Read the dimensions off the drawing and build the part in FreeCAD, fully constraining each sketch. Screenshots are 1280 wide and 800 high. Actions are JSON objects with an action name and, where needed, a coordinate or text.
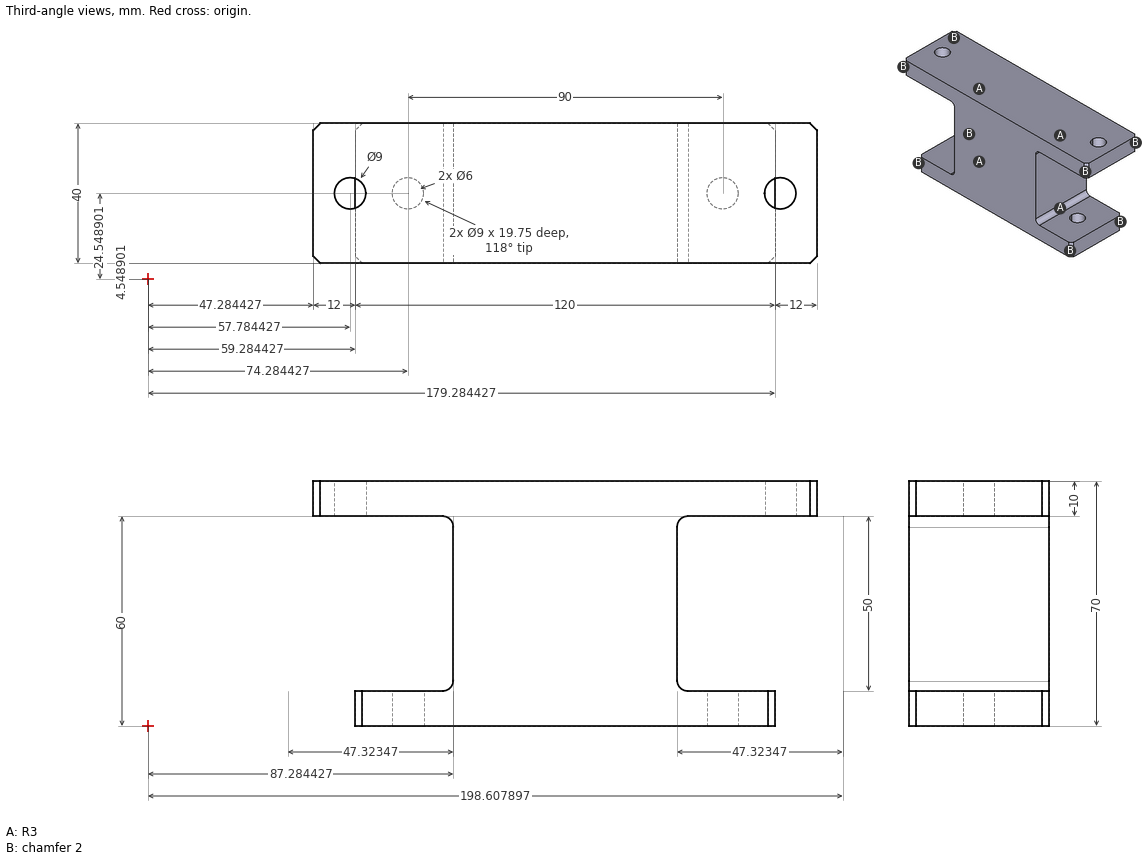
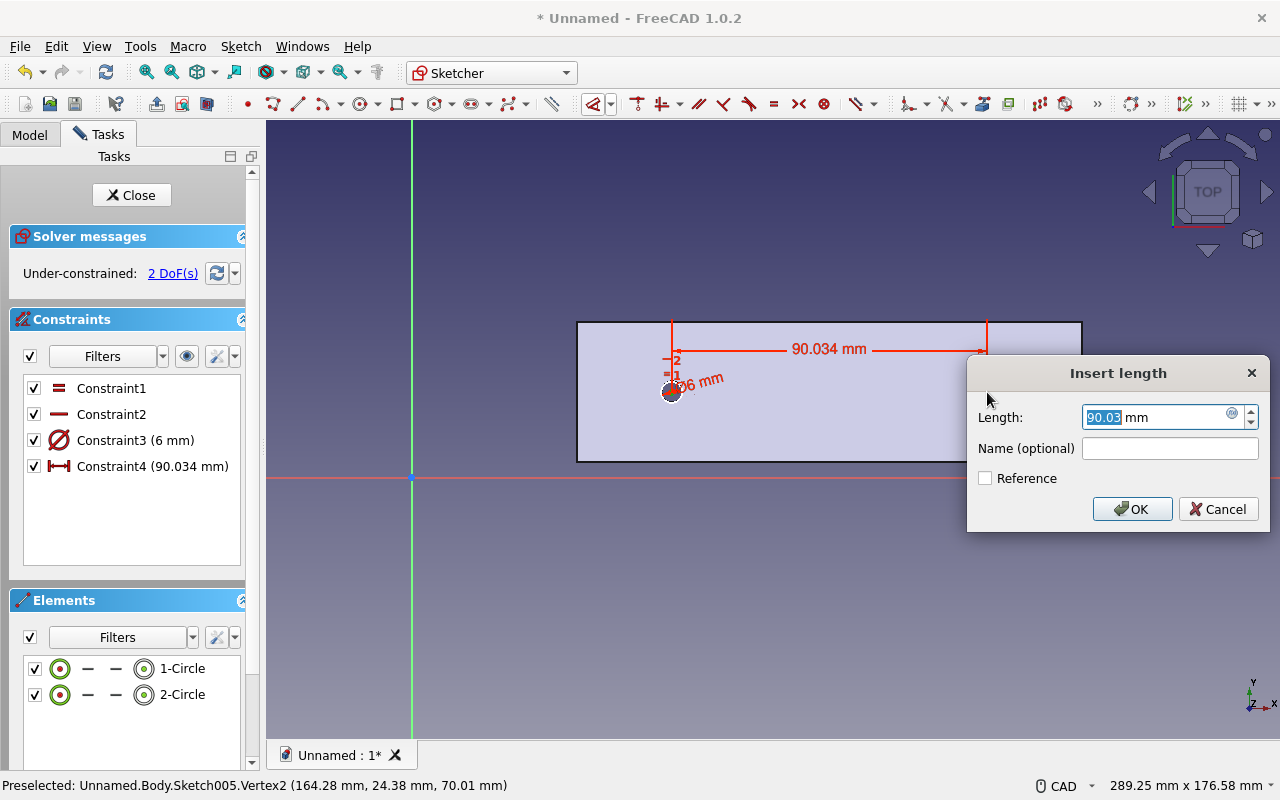
{"action": "type", "text": "90"}
{"action": "key", "text": "Return"}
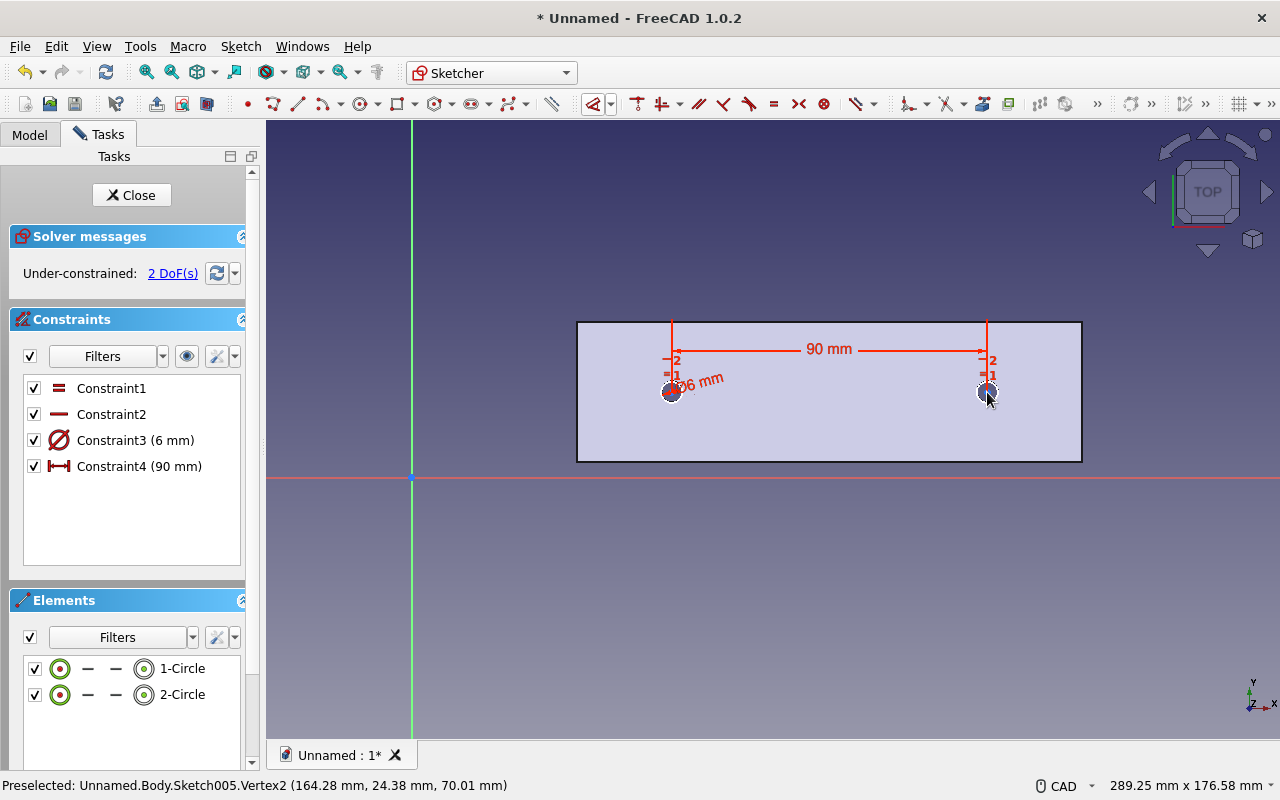
{"action": "left_click", "coordinate": [672, 392]}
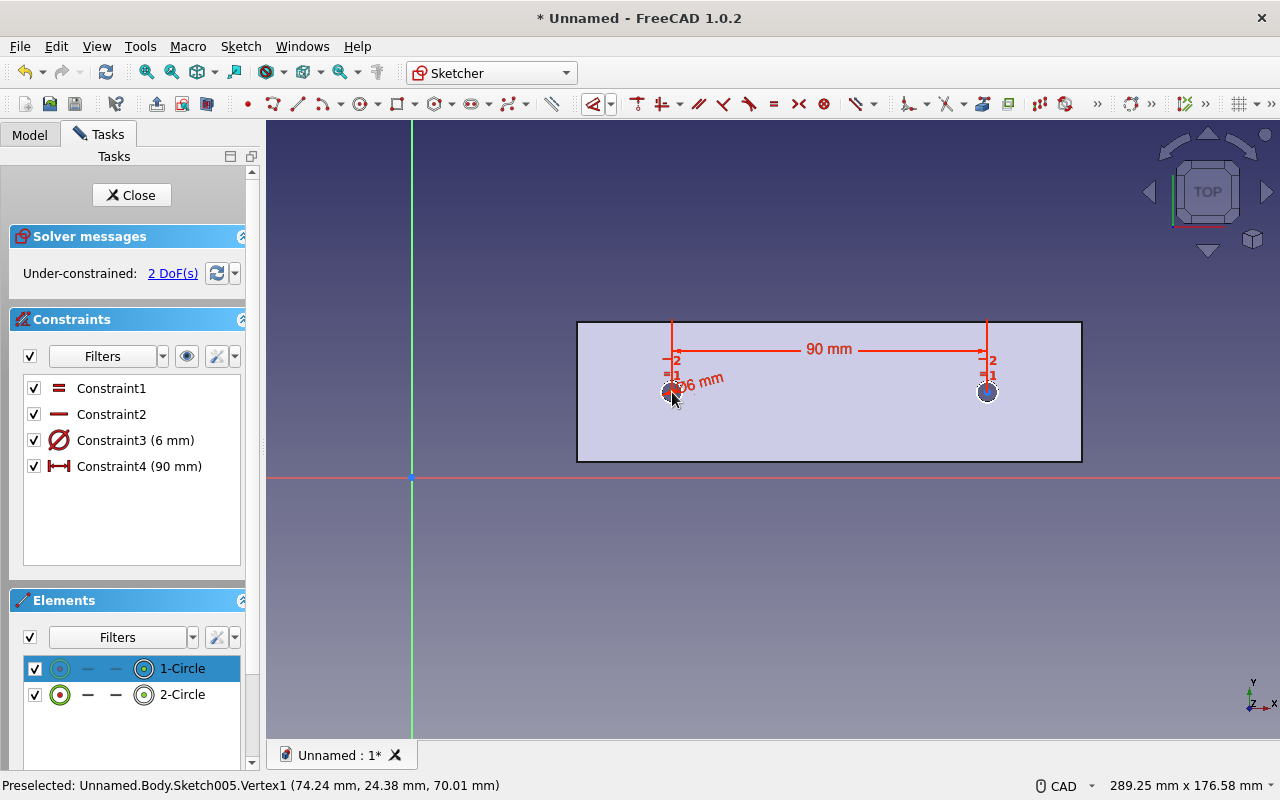
{"action": "key", "text": "l"}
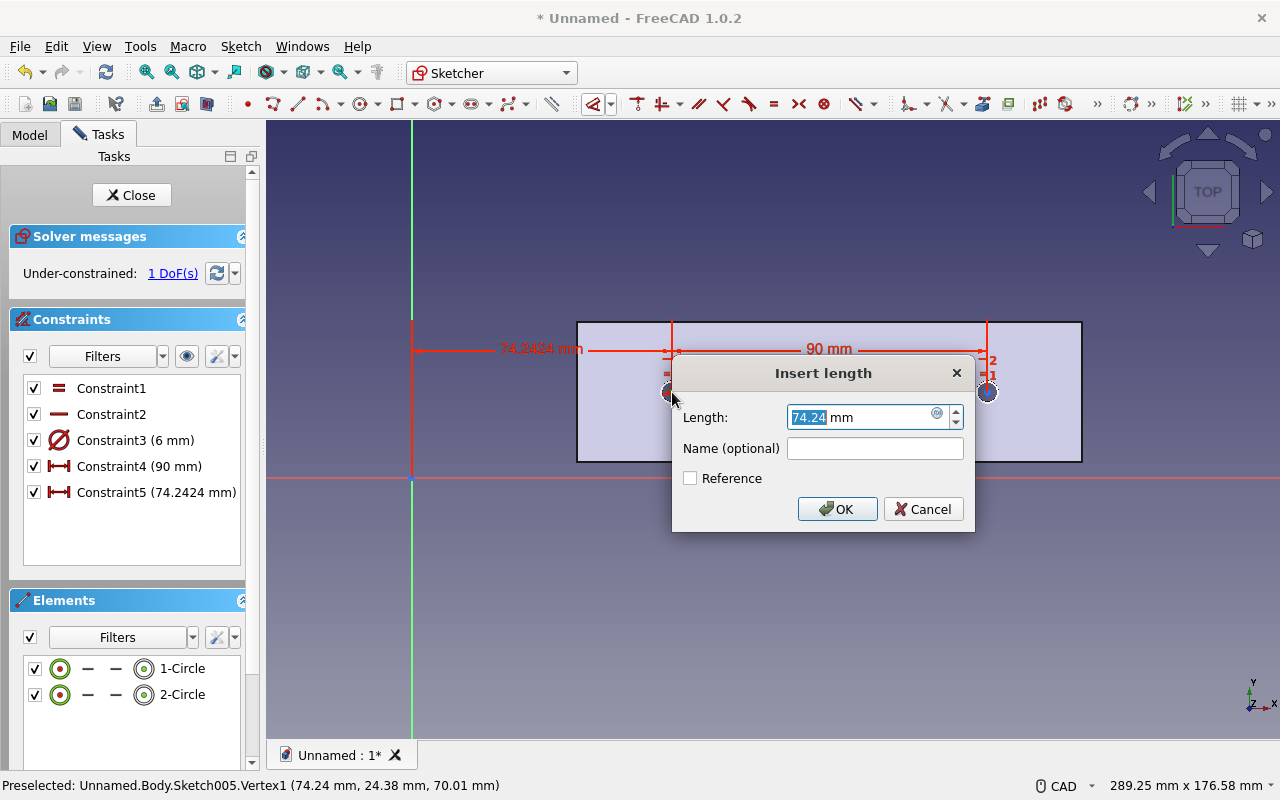
{"action": "type", "text": "74.284427"}
{"action": "key", "text": "Return"}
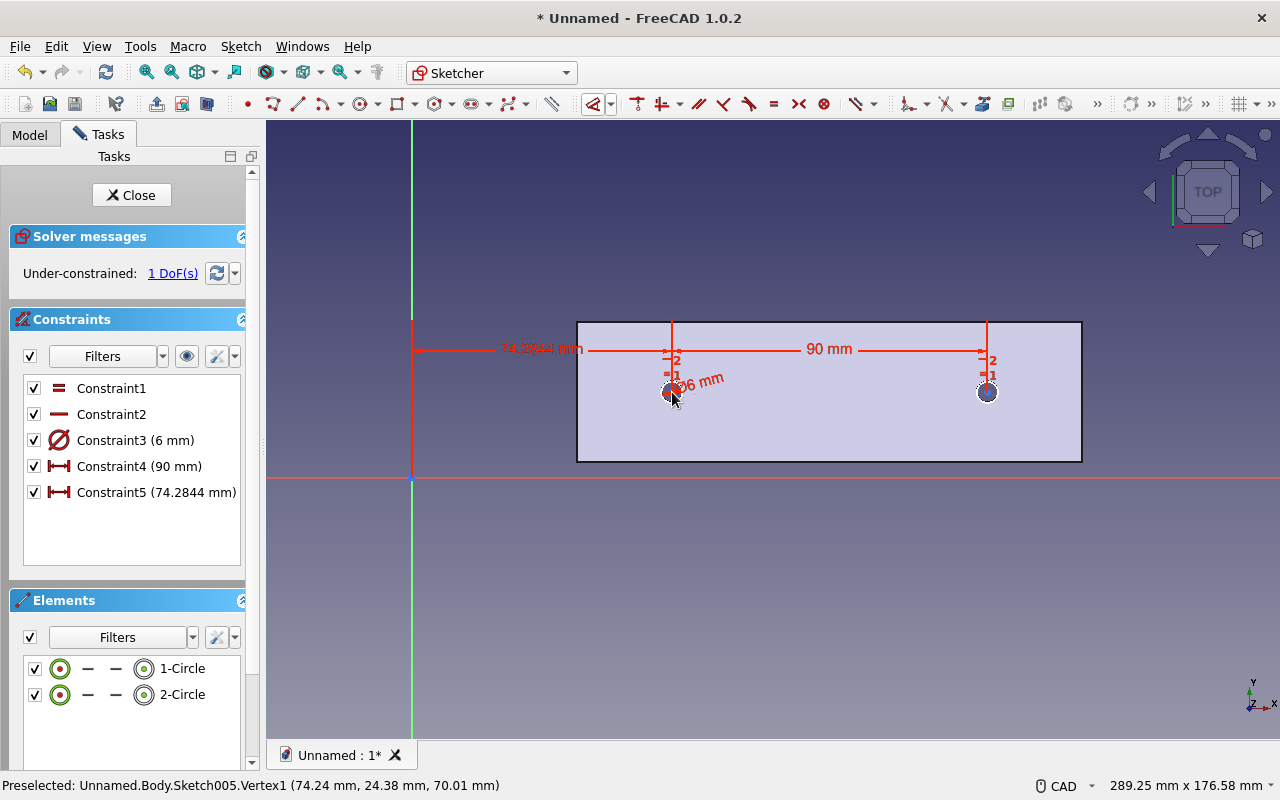
{"action": "left_click", "coordinate": [672, 392]}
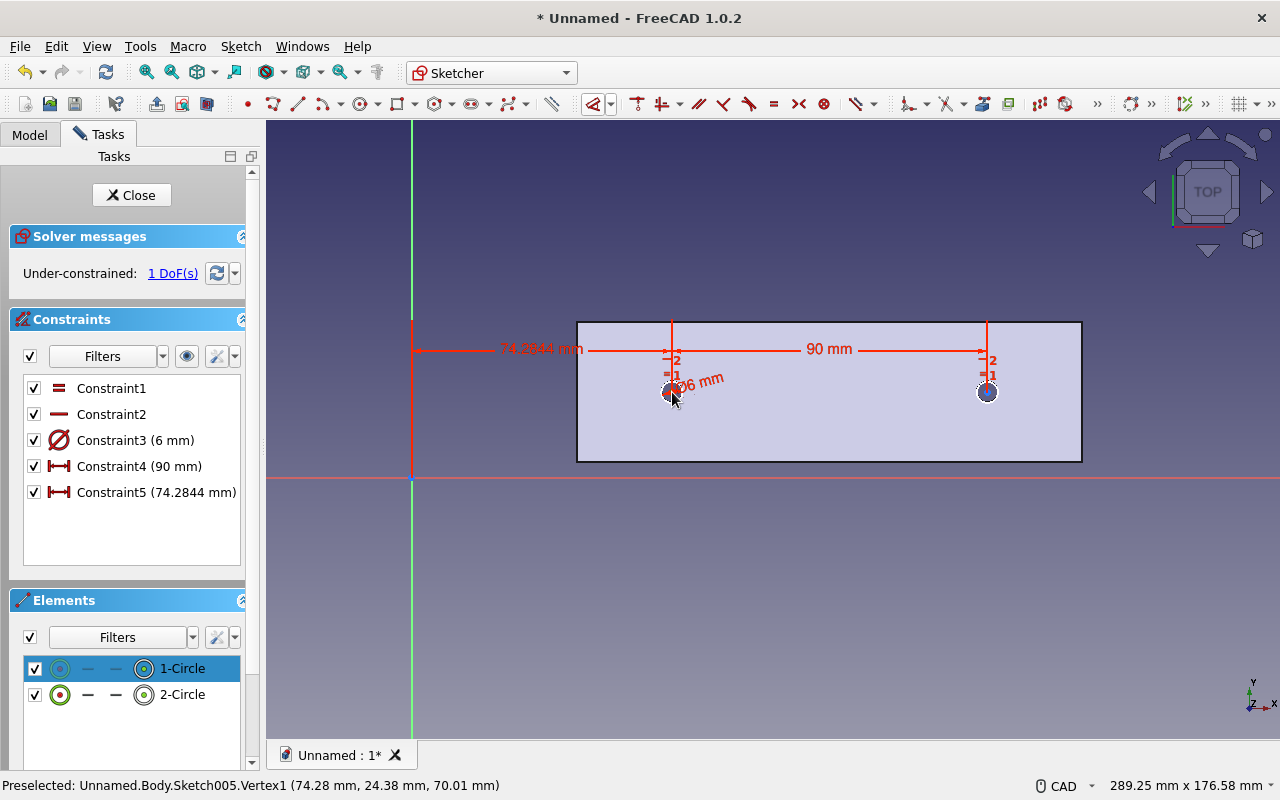
{"action": "key", "text": "i"}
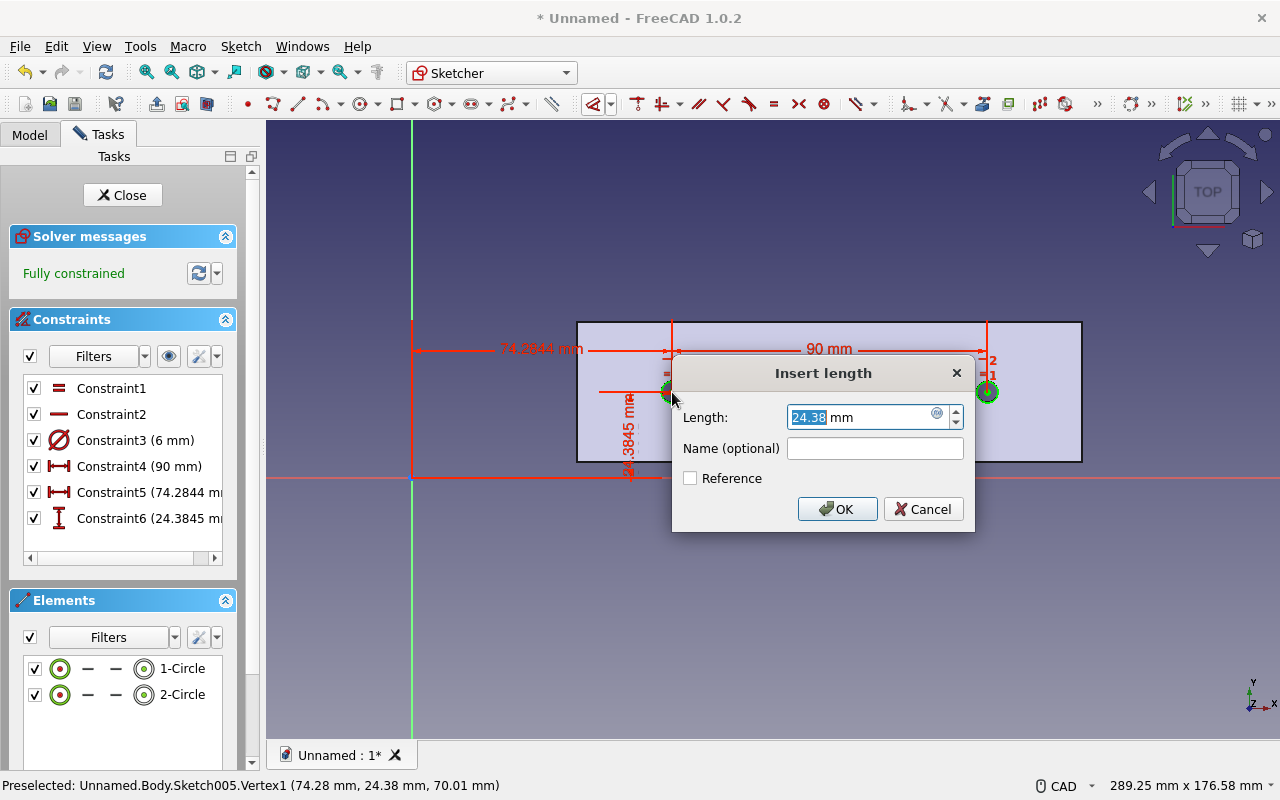
{"action": "type", "text": "24.548901"}
{"action": "key", "text": "Return"}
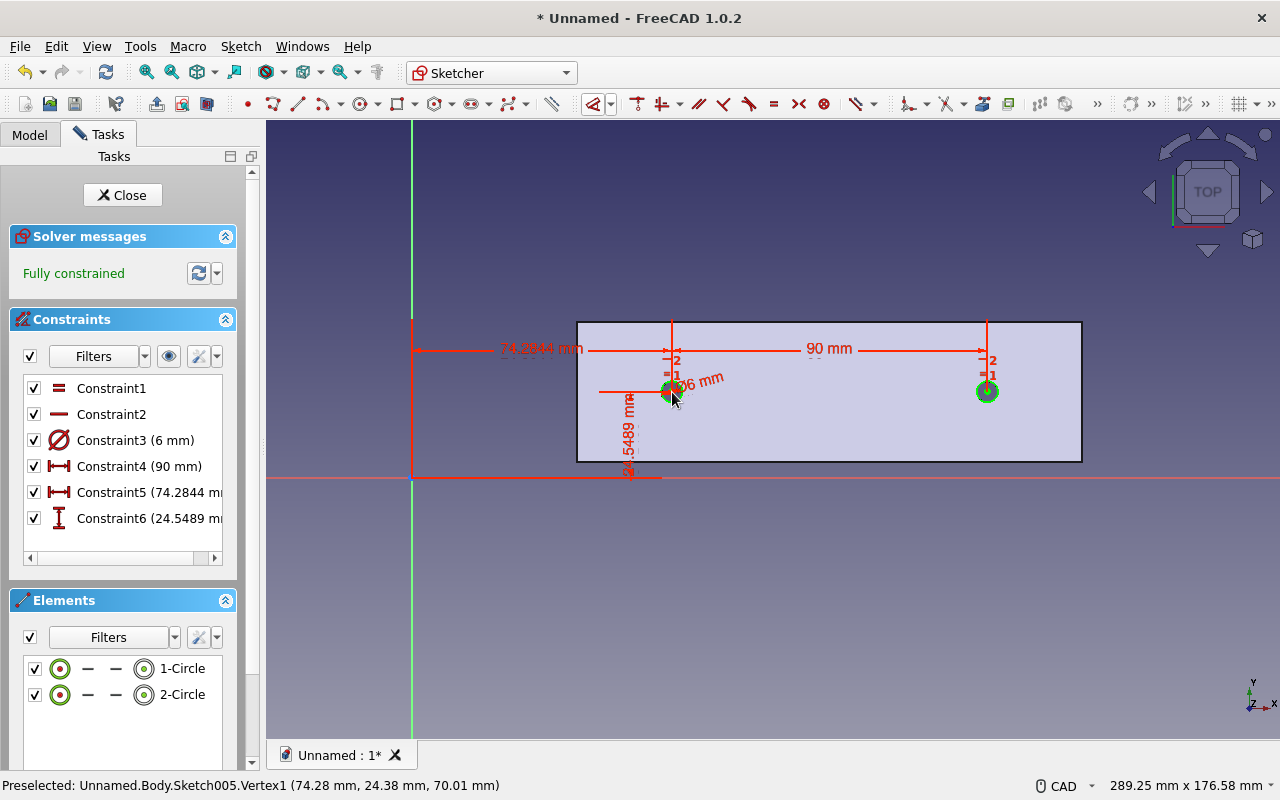
{"action": "left_click", "coordinate": [123, 195]}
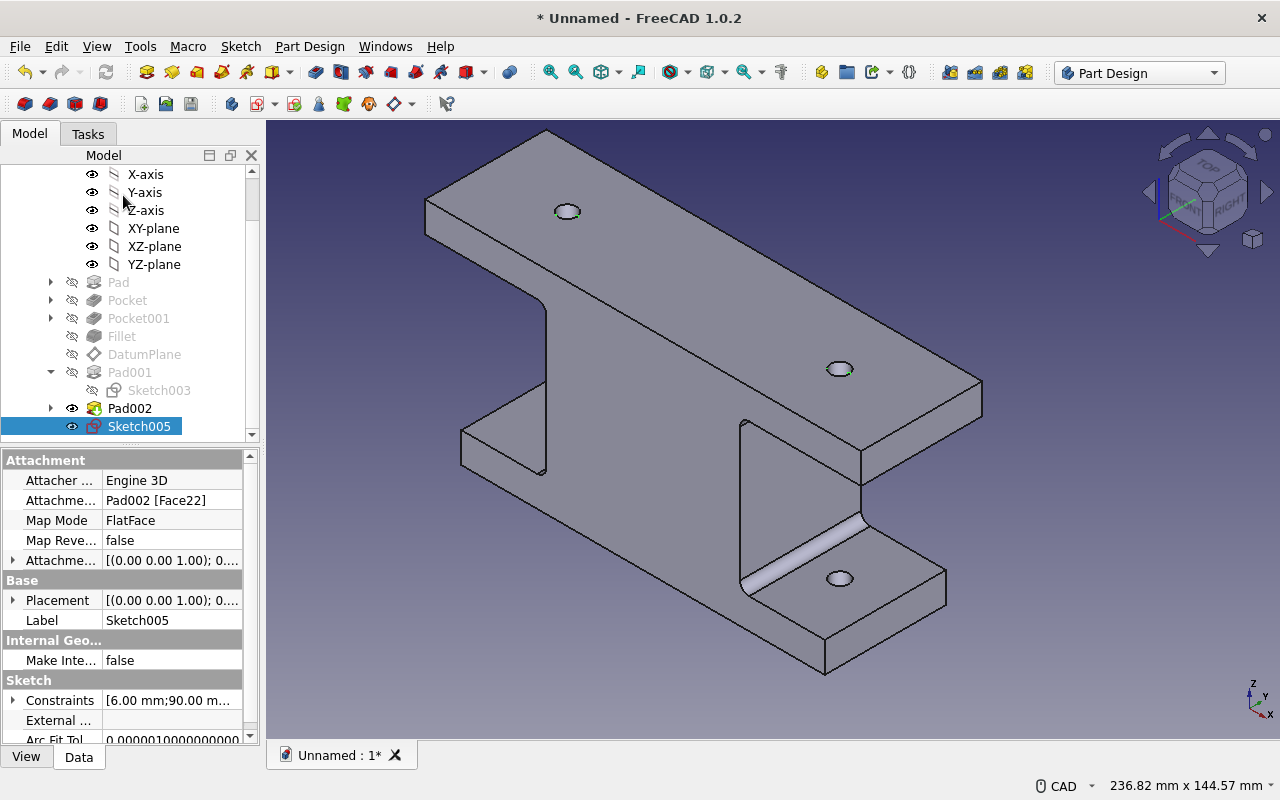
{"action": "left_click", "coordinate": [147, 72]}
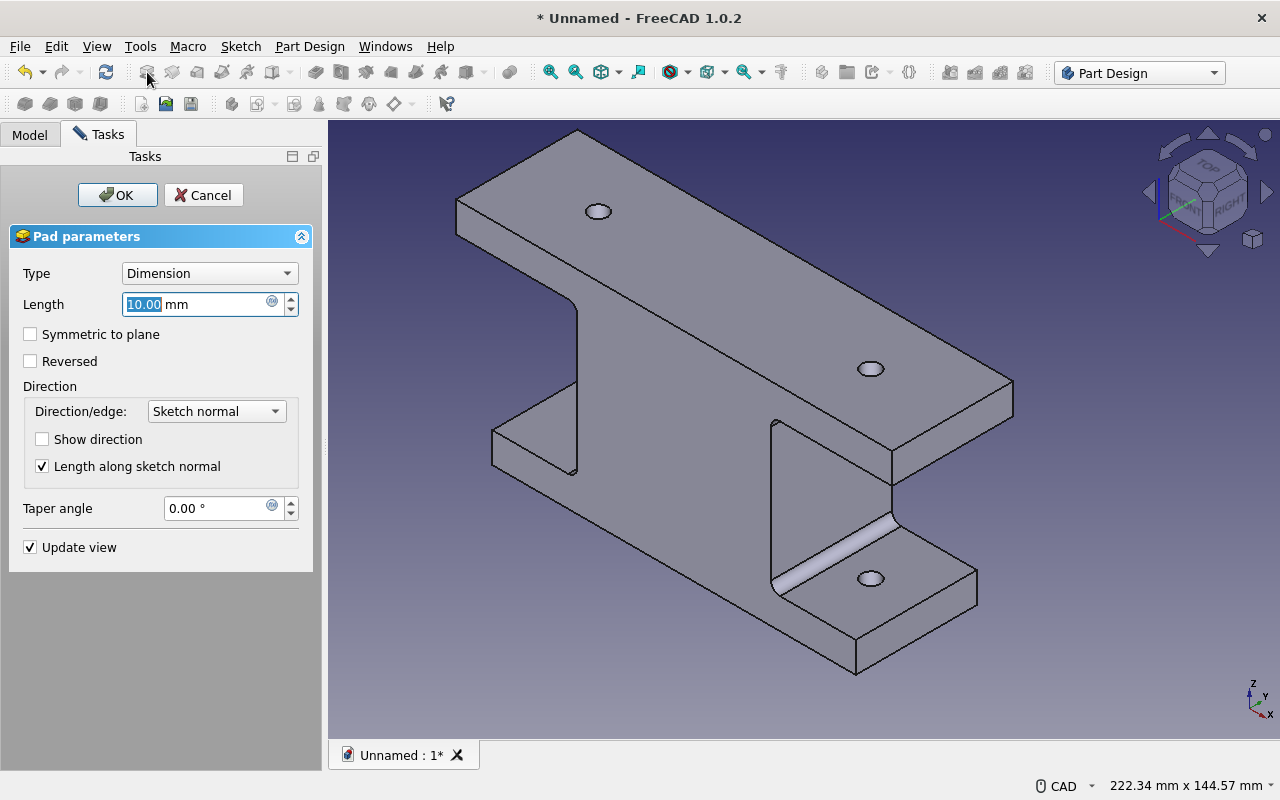
{"action": "type", "text": "10"}
{"action": "key", "text": "Tab"}